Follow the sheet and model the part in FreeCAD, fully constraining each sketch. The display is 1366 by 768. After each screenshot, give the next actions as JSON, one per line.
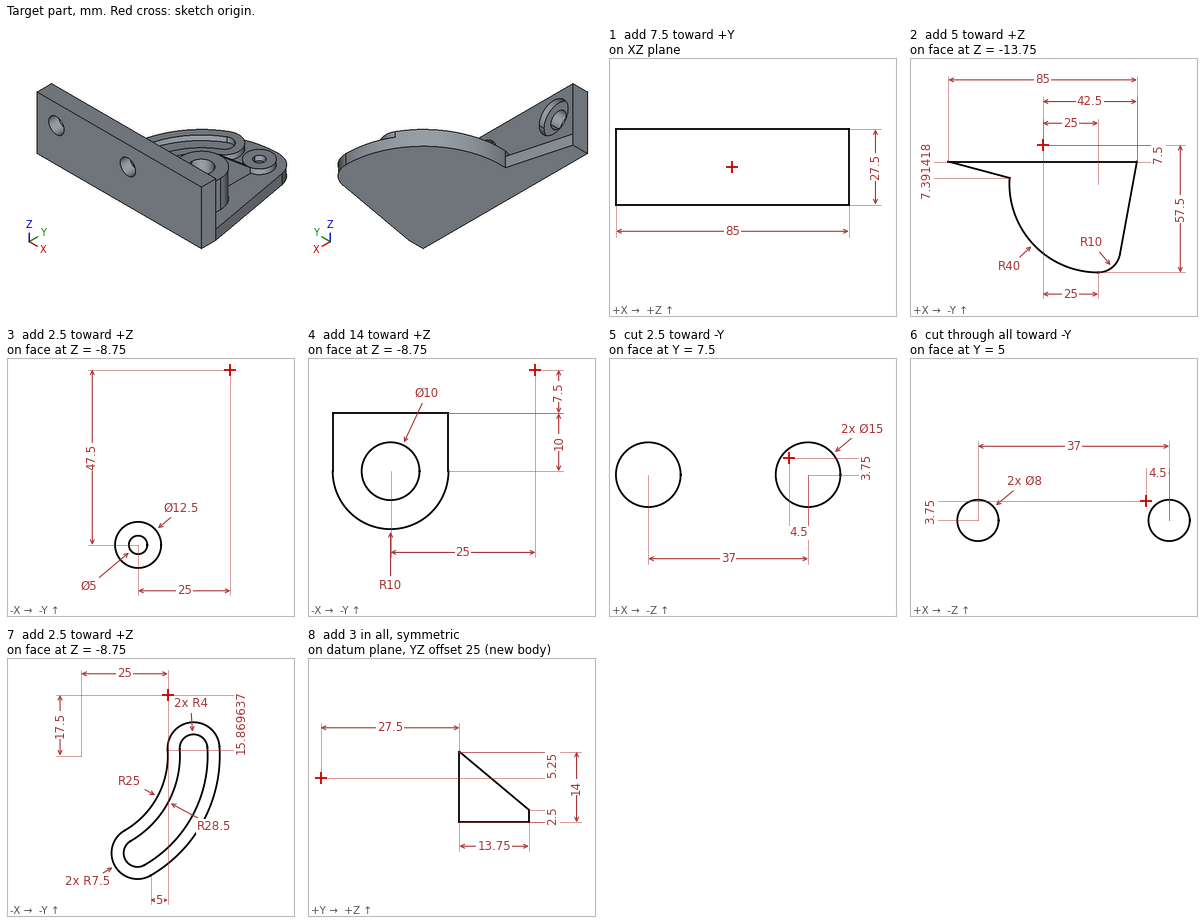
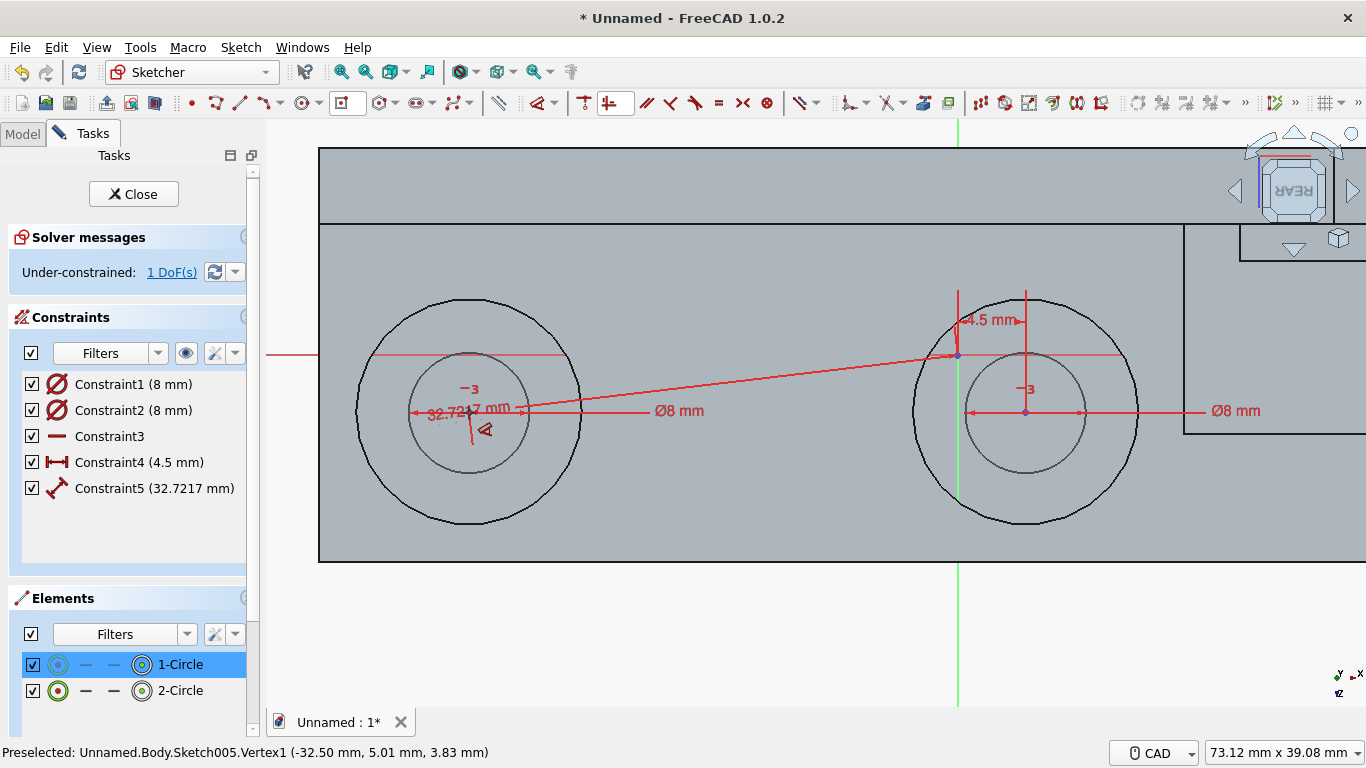
{"action": "left_click", "coordinate": [1026, 413]}
{"action": "left_click", "coordinate": [747, 447]}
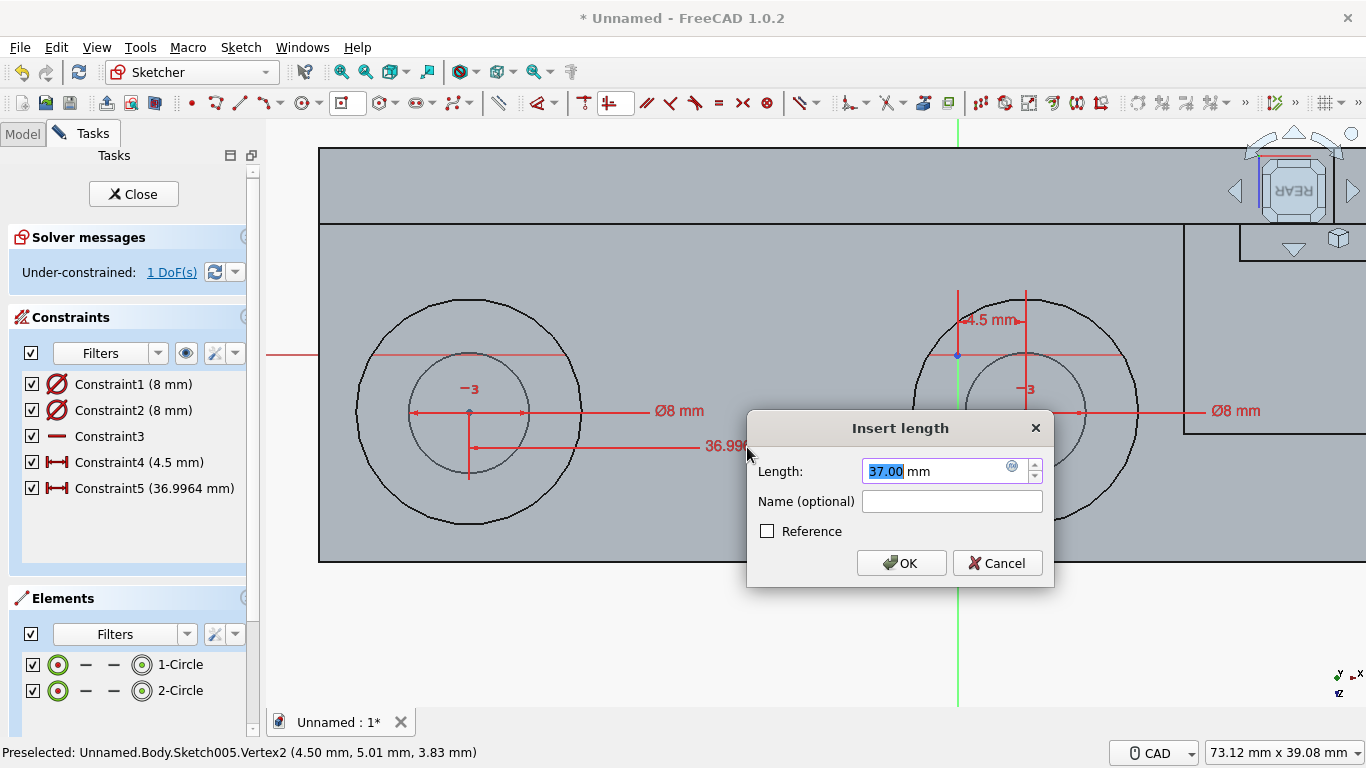
{"action": "type", "text": "37"}
{"action": "key", "text": "Return"}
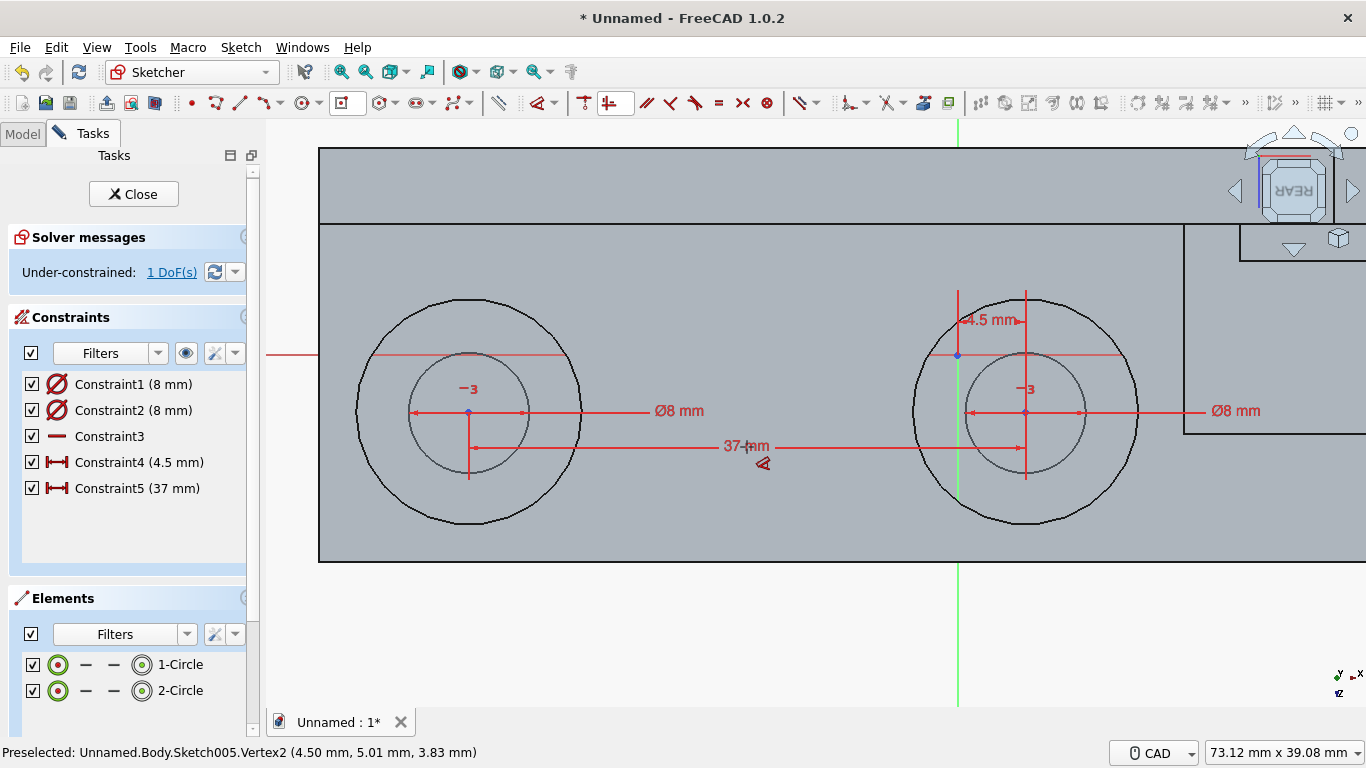
{"action": "left_click", "coordinate": [469, 413]}
{"action": "left_click", "coordinate": [435, 384]}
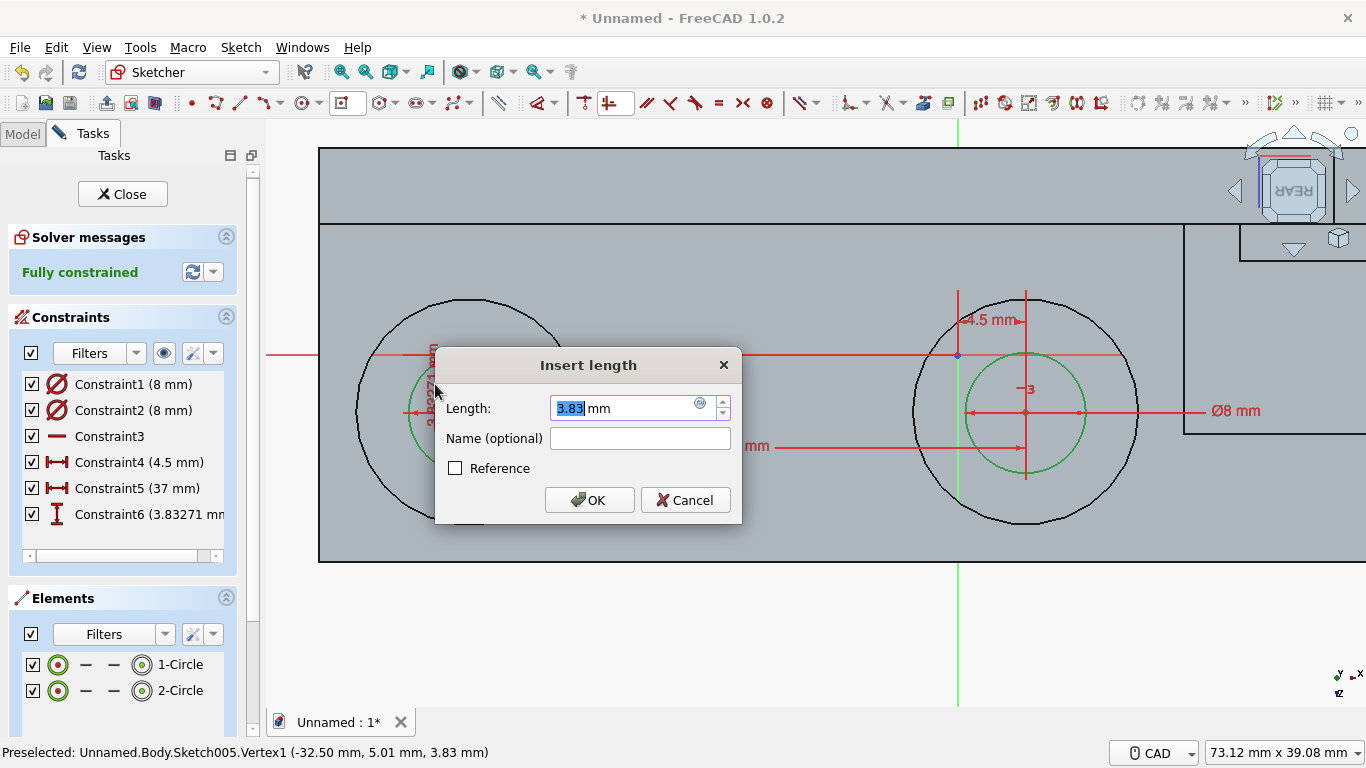
{"action": "type", "text": "3.75"}
{"action": "key", "text": "Return"}
{"action": "key", "text": "Escape"}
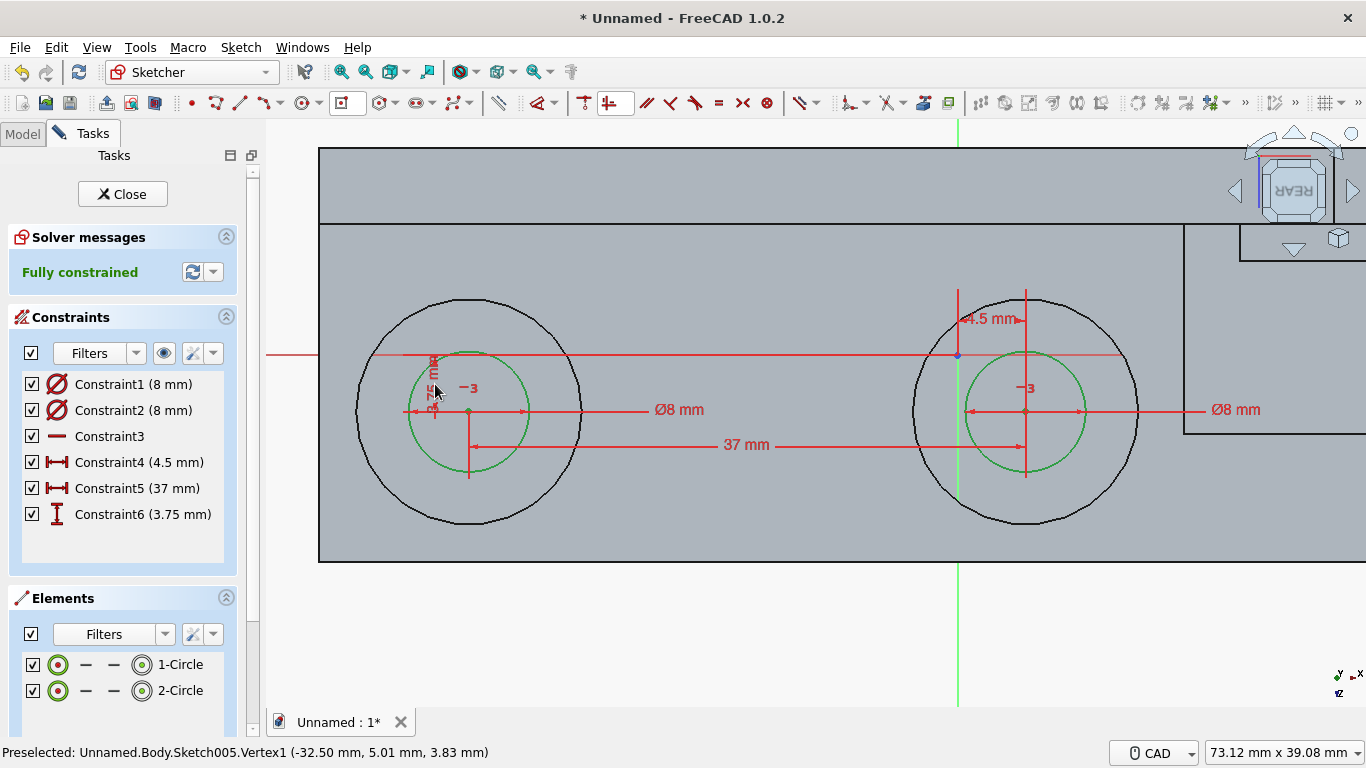
{"action": "left_click", "coordinate": [123, 194]}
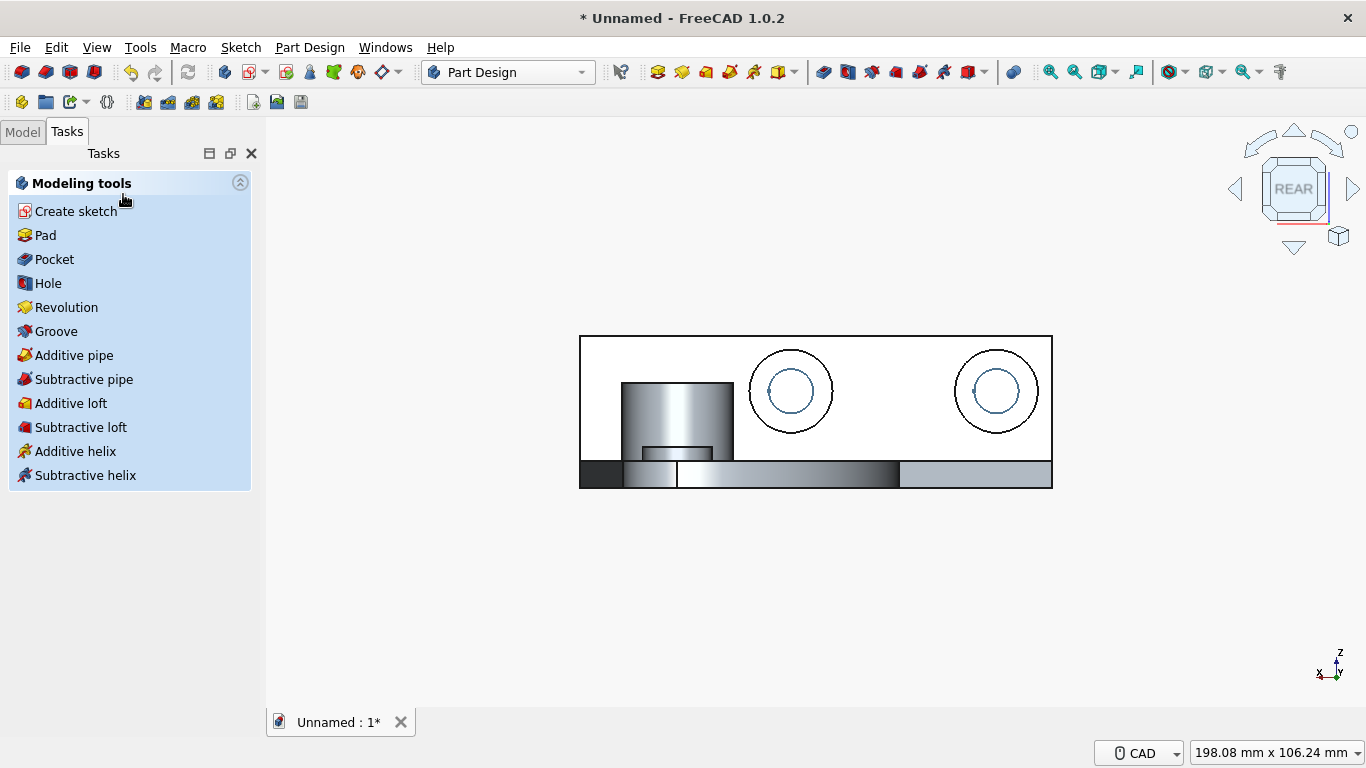
{"action": "left_click", "coordinate": [824, 72]}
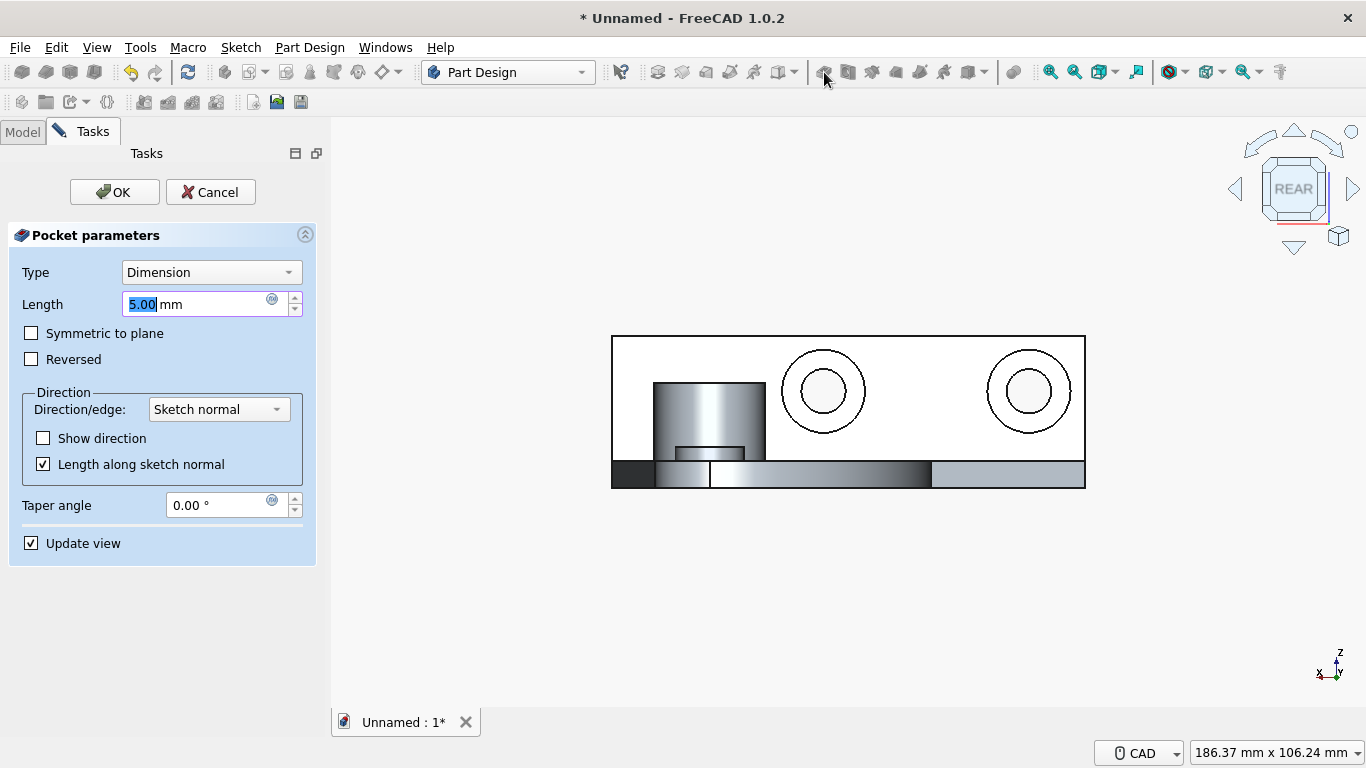
{"action": "left_click", "coordinate": [212, 272]}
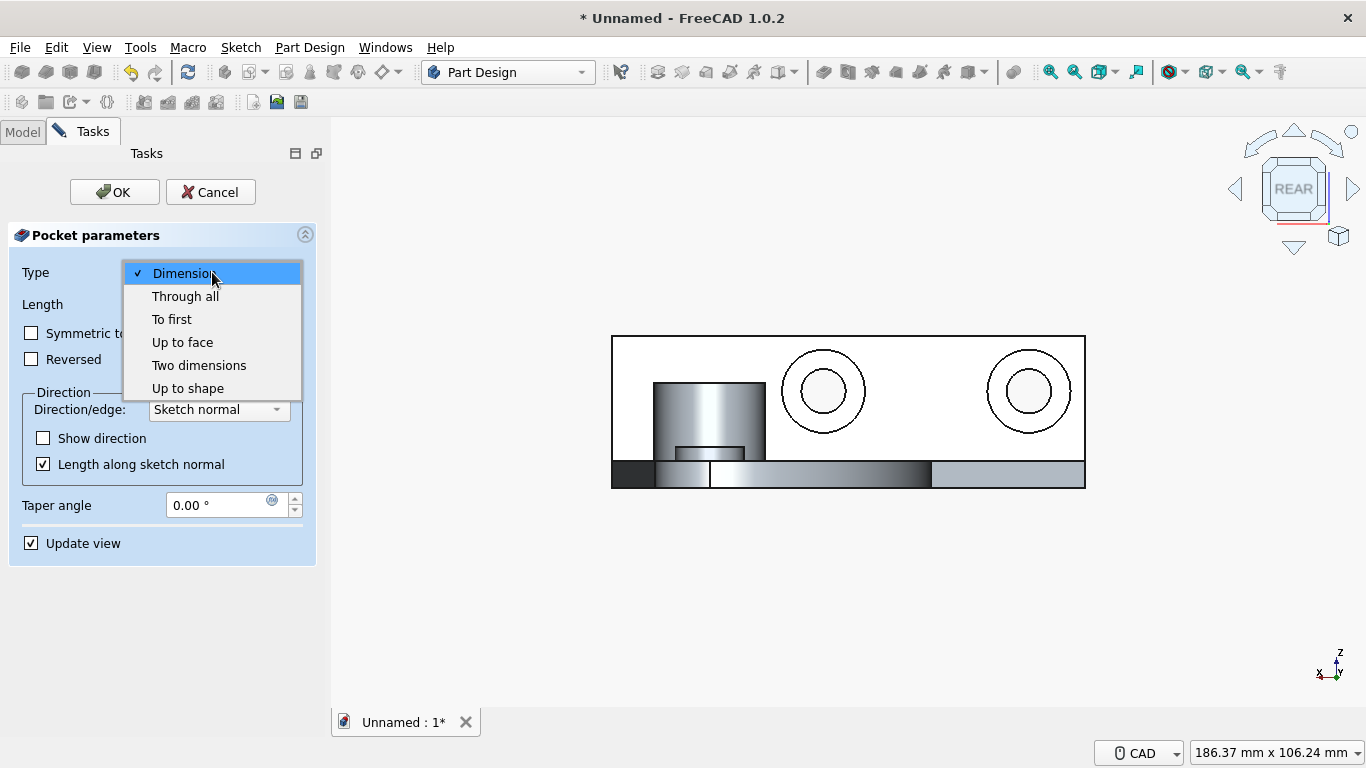
{"action": "left_click", "coordinate": [212, 296]}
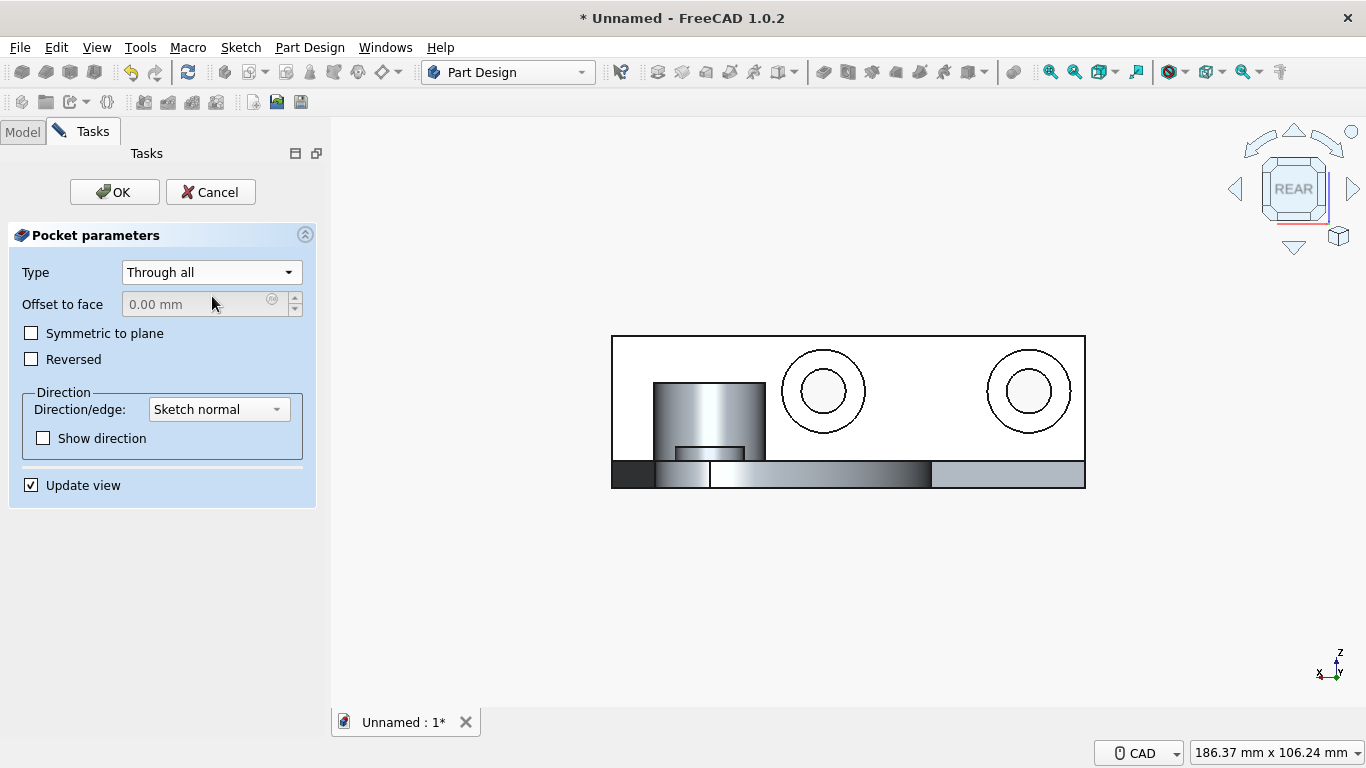
{"action": "left_click", "coordinate": [115, 192]}